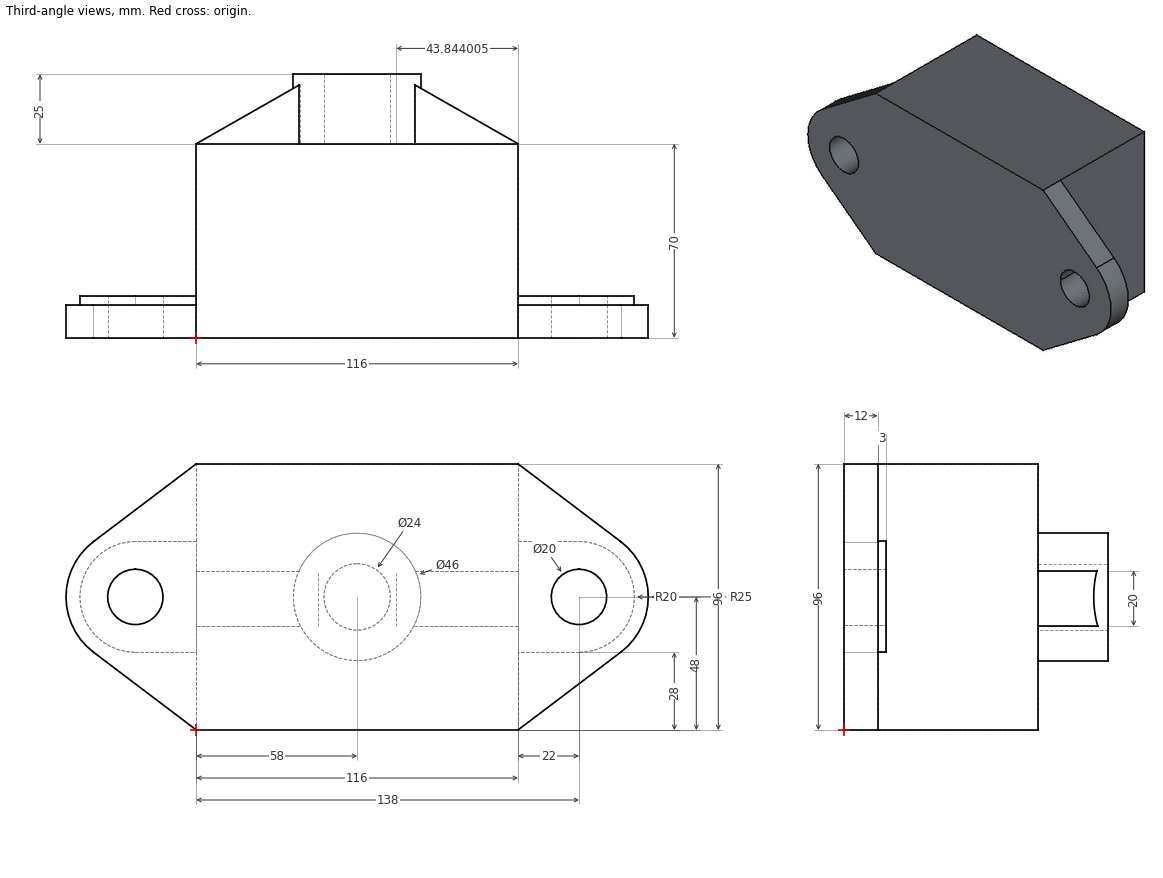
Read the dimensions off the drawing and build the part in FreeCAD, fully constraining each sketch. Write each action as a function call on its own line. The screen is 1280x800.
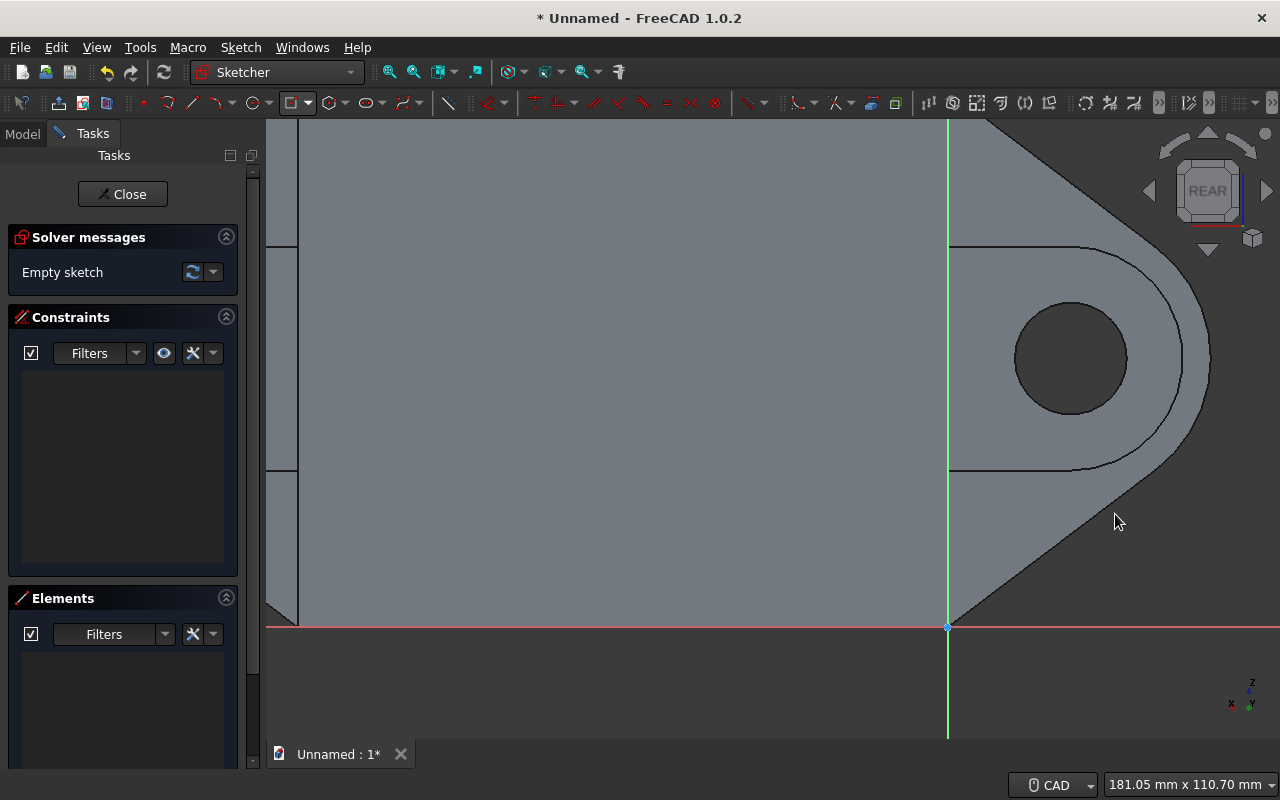
click(254, 104)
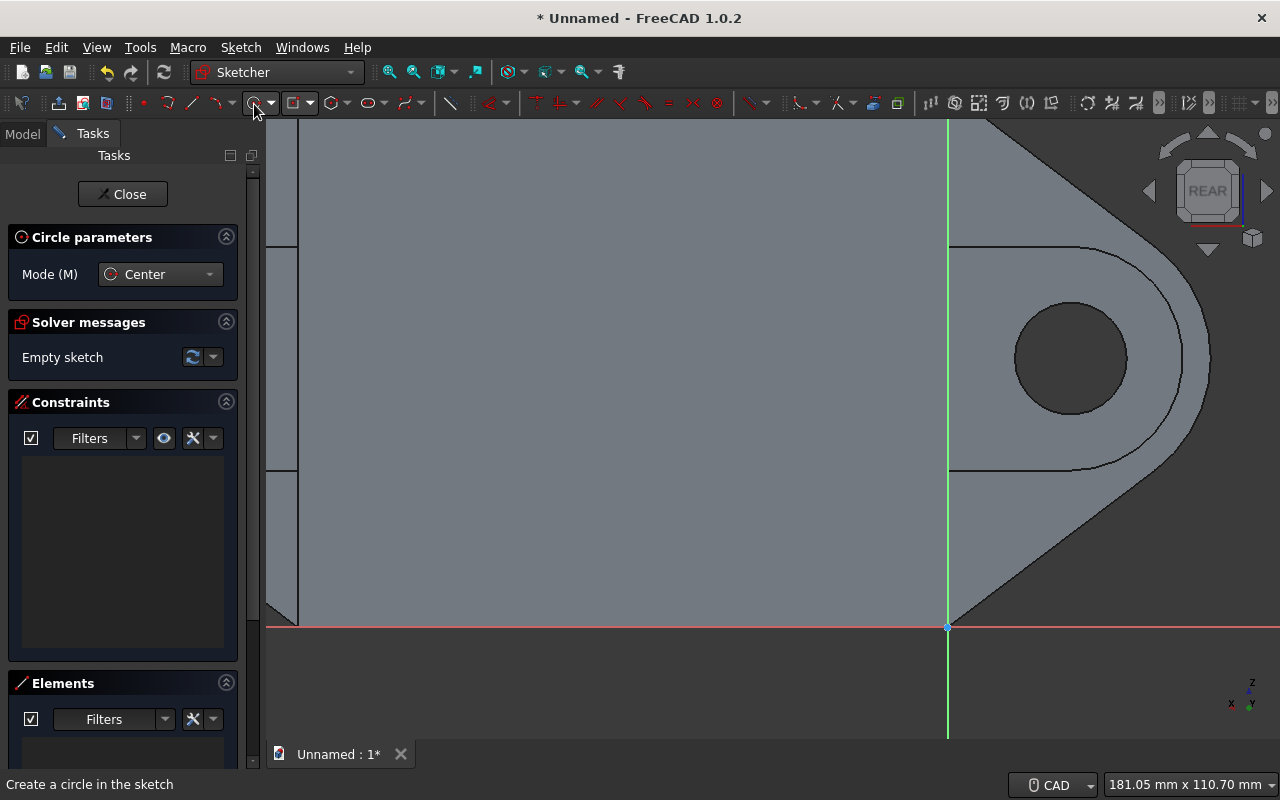
click(623, 359)
move(714, 268)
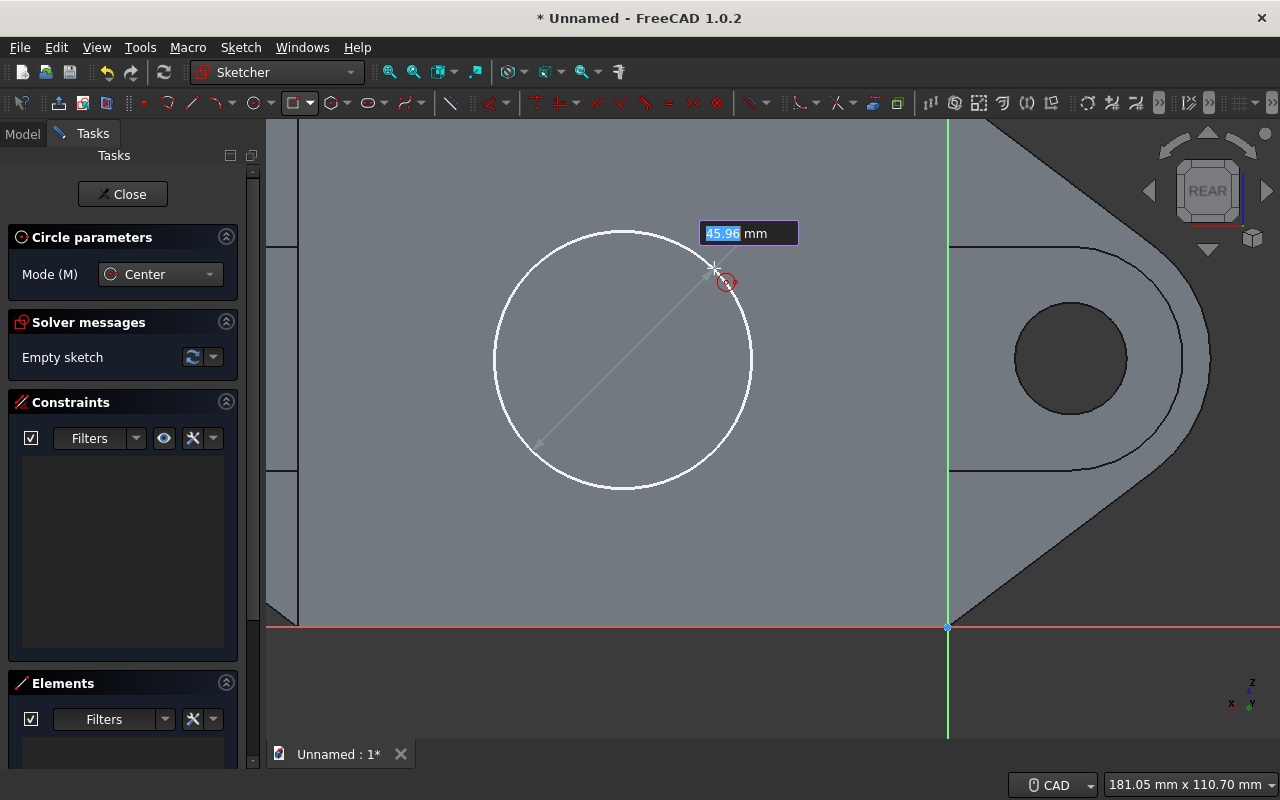
text(46)
key(Return)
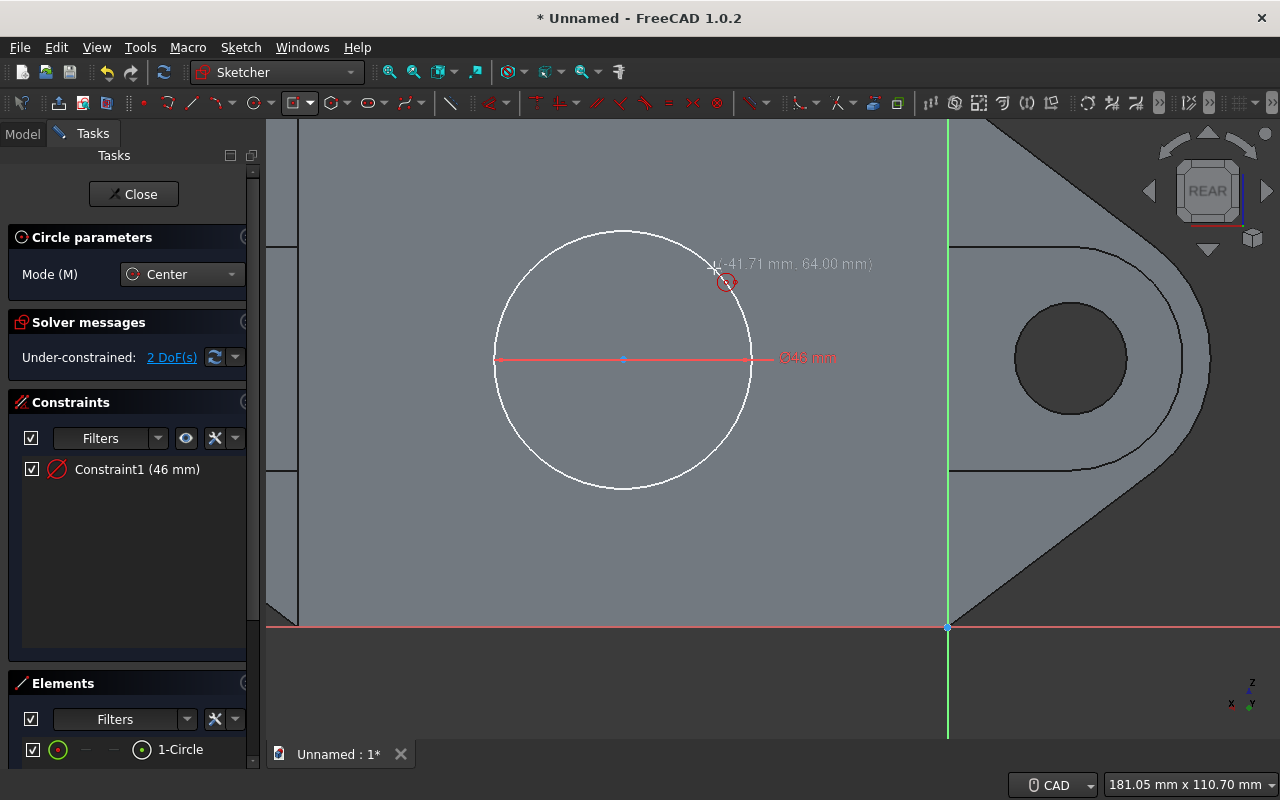
click(623, 360)
move(670, 311)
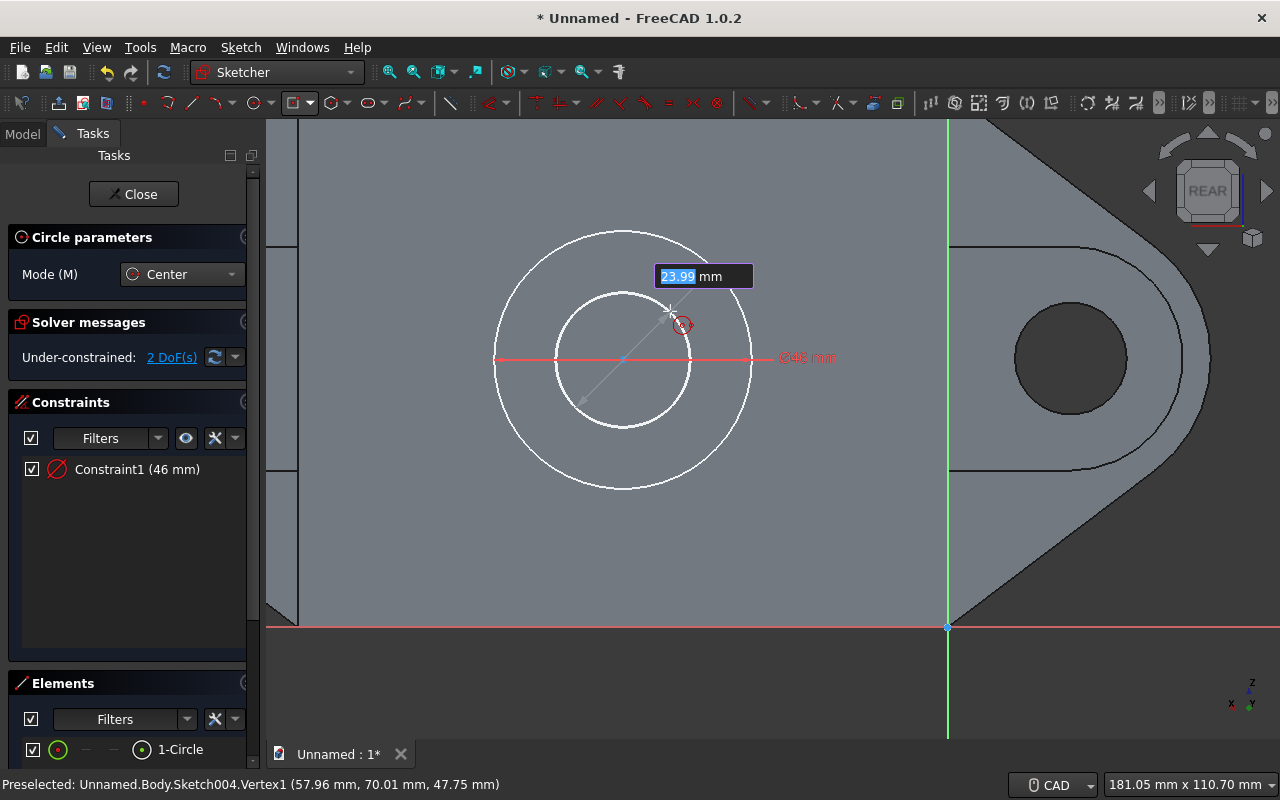
text(24)
key(Return)
key(Escape)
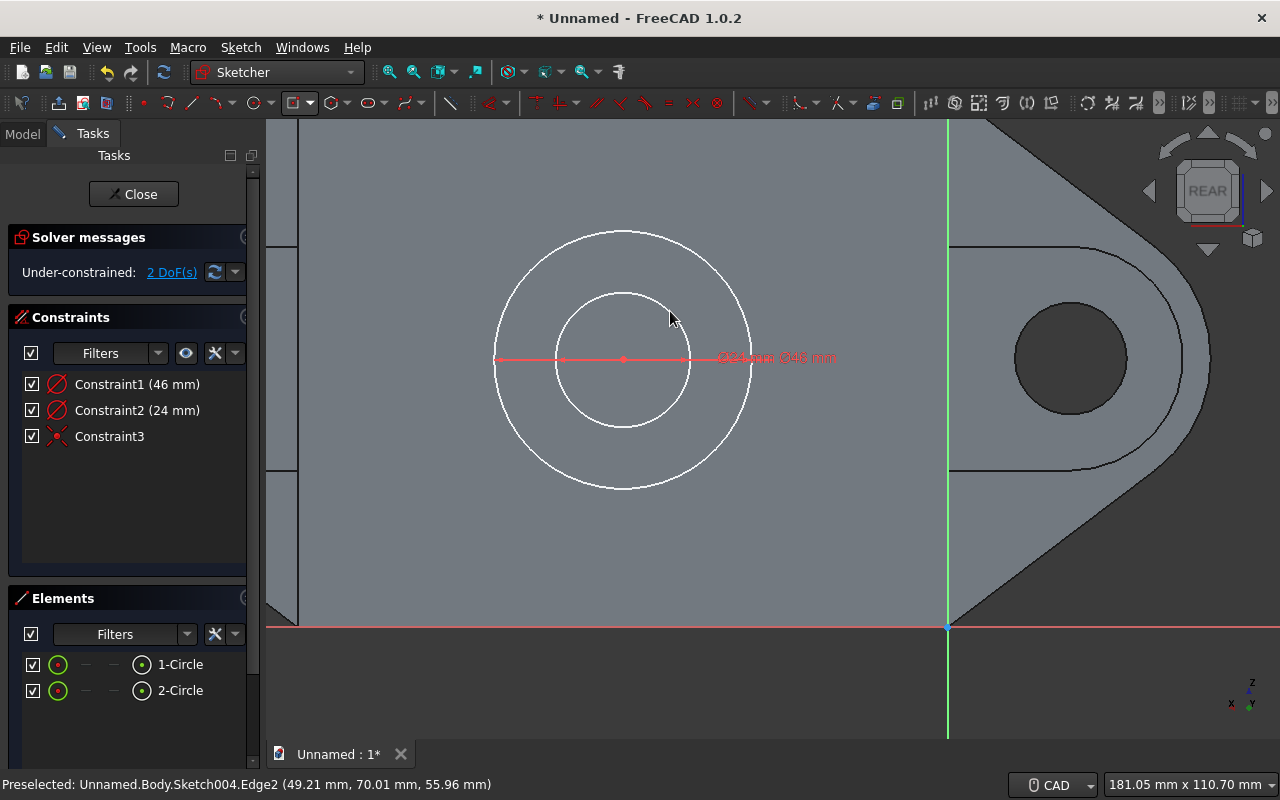
click(490, 104)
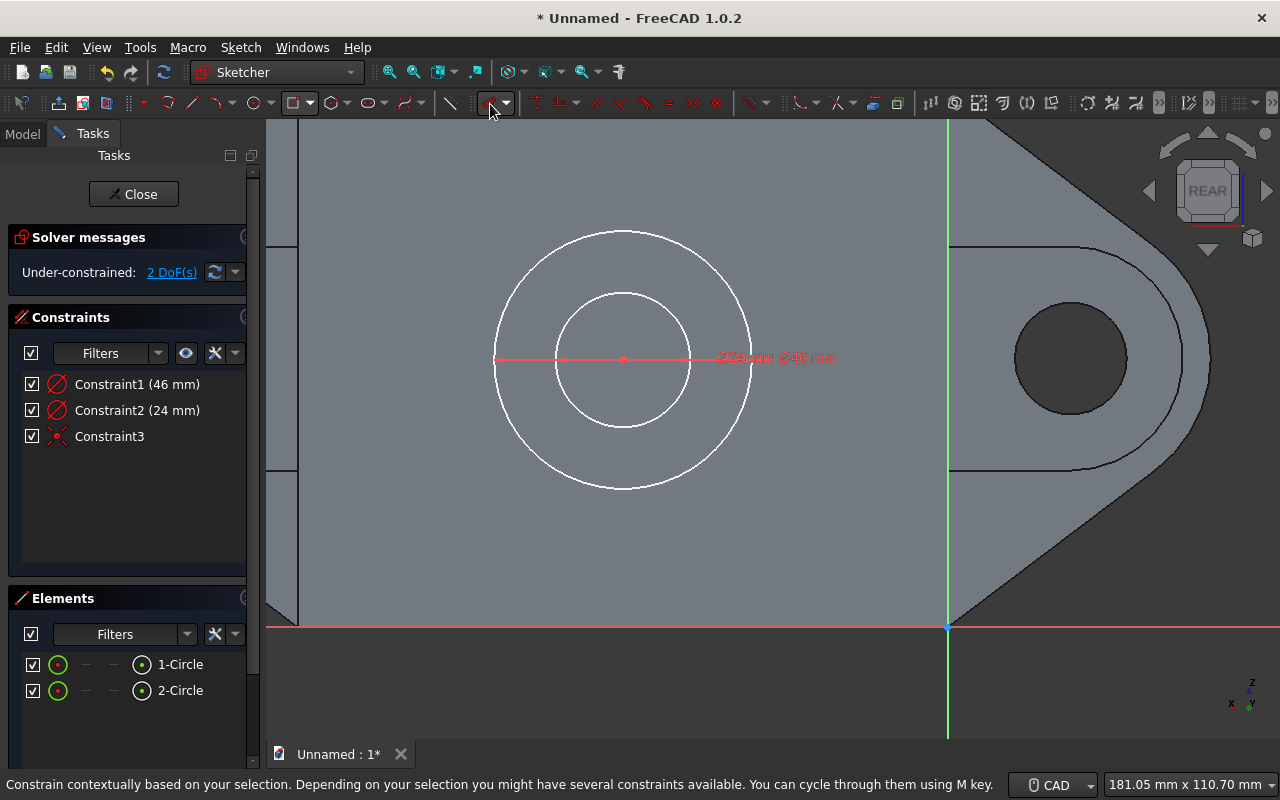
click(623, 360)
click(785, 661)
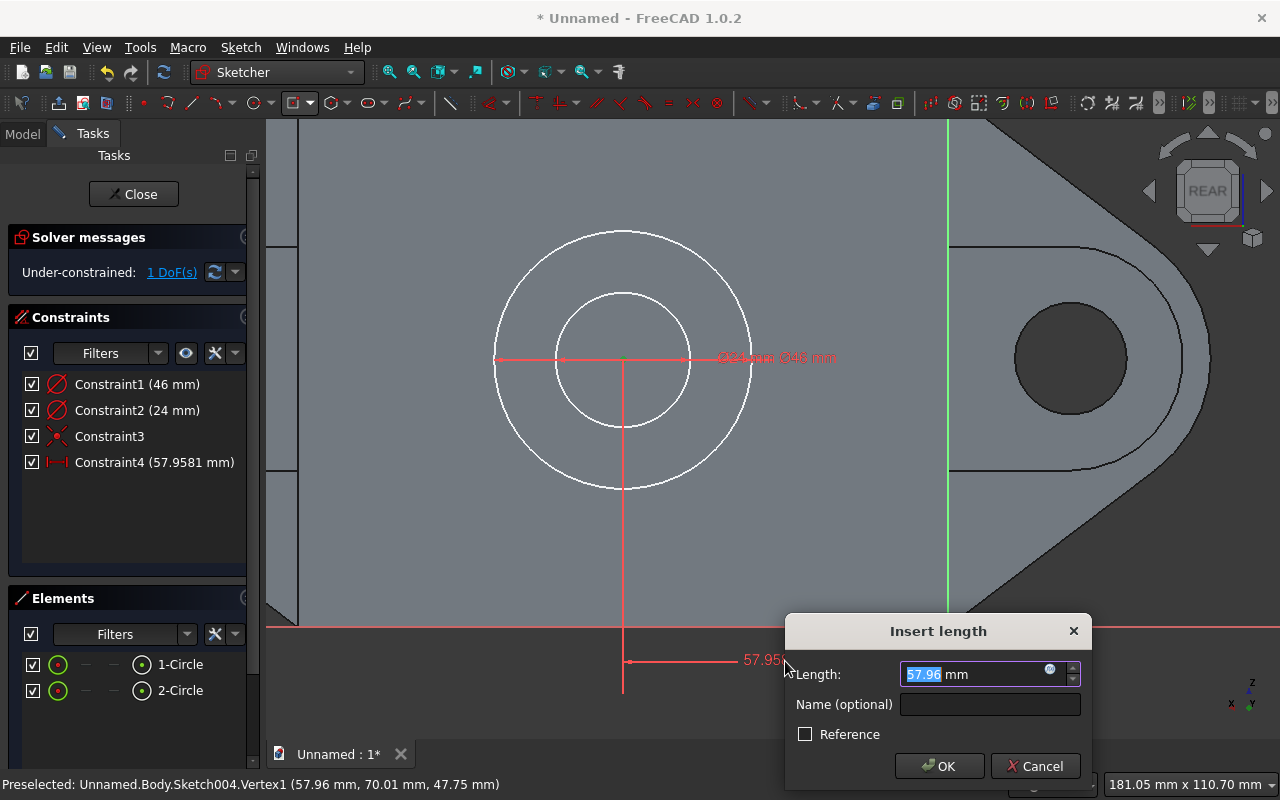
text(58)
key(Return)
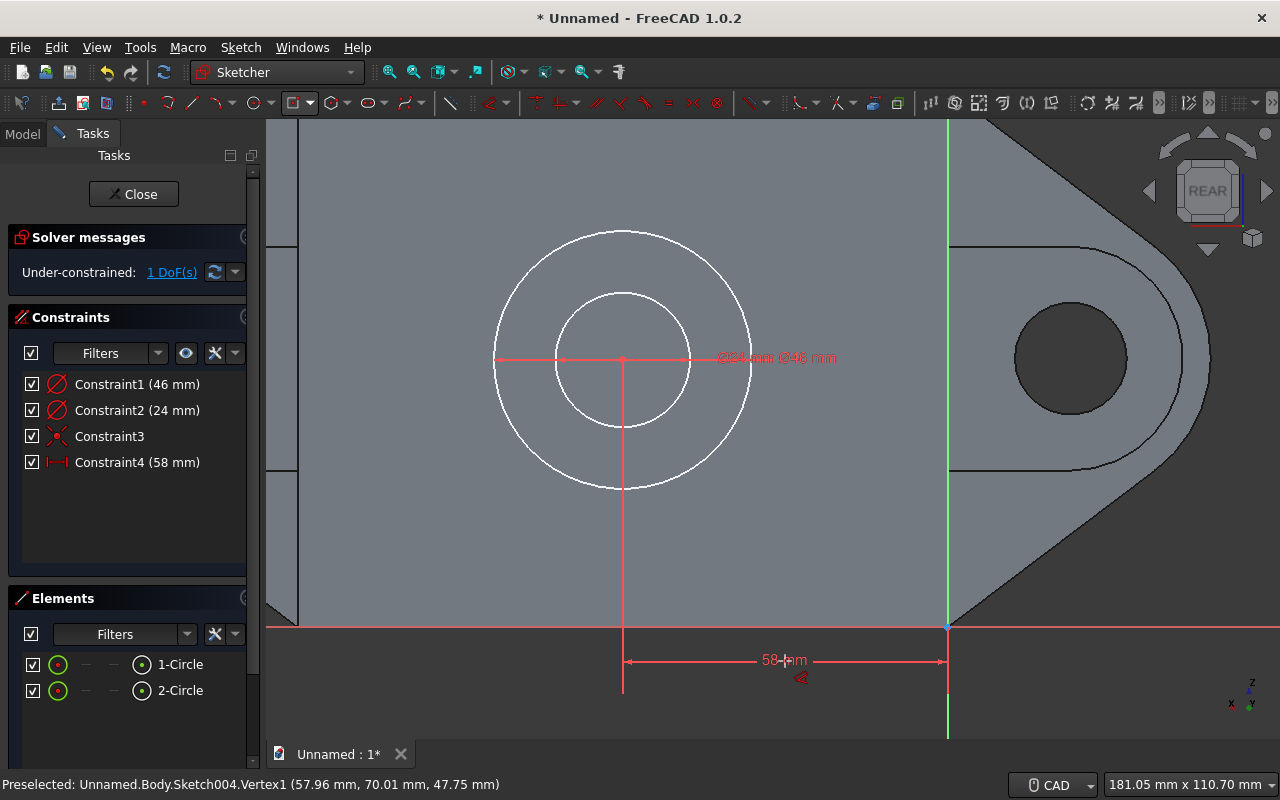
click(623, 360)
click(982, 494)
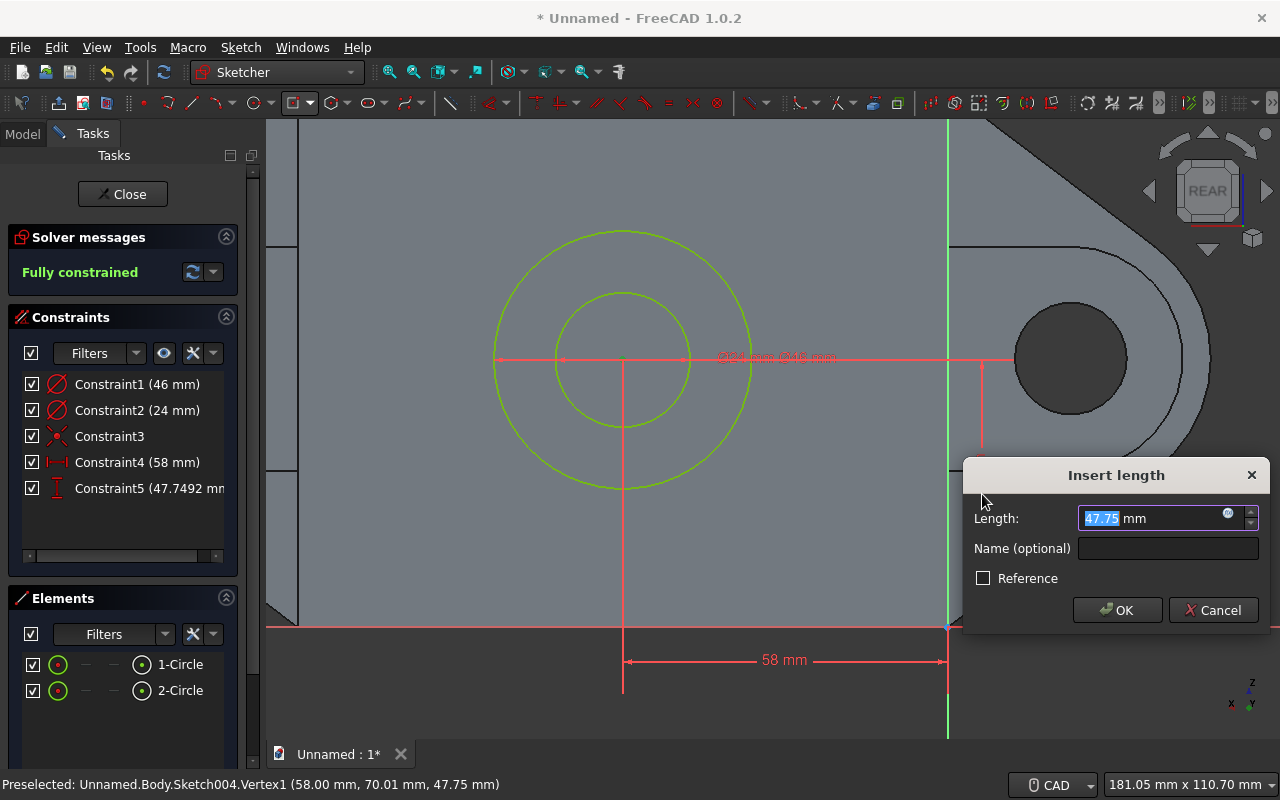
text(48)
key(Return)
key(Escape)